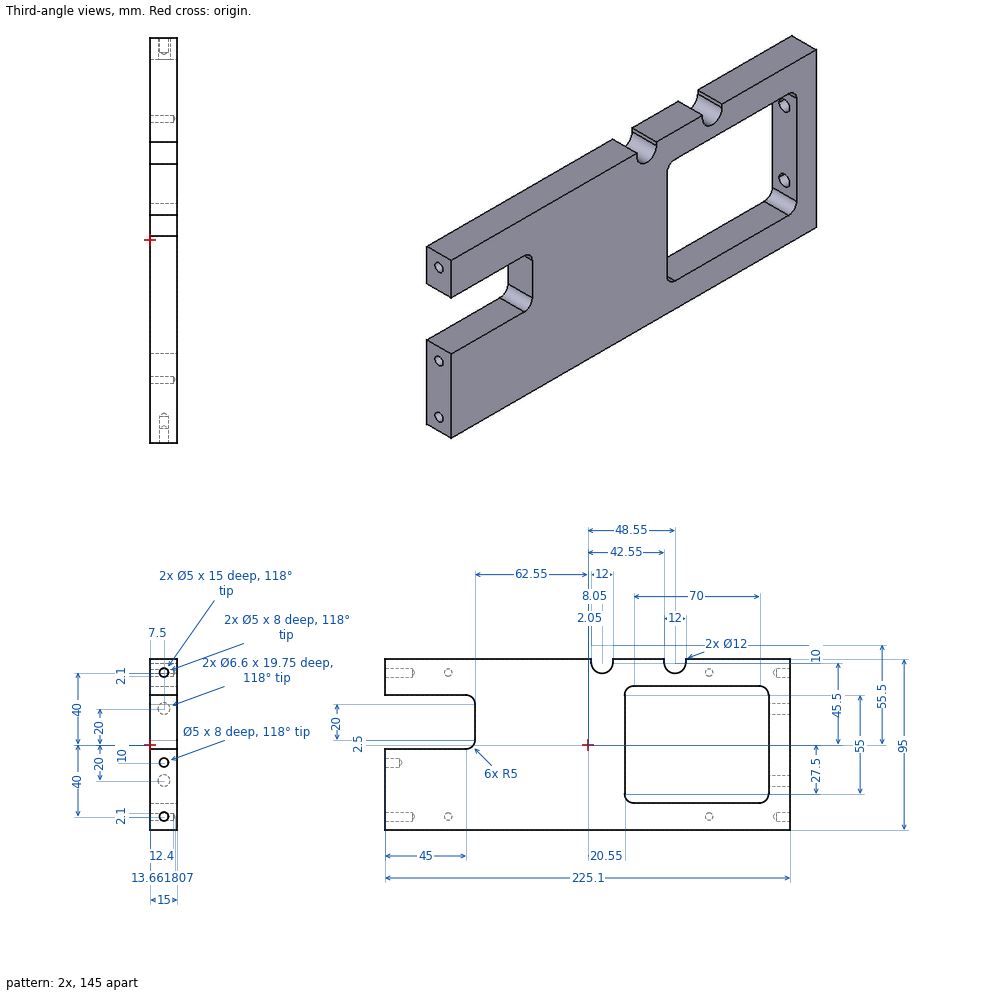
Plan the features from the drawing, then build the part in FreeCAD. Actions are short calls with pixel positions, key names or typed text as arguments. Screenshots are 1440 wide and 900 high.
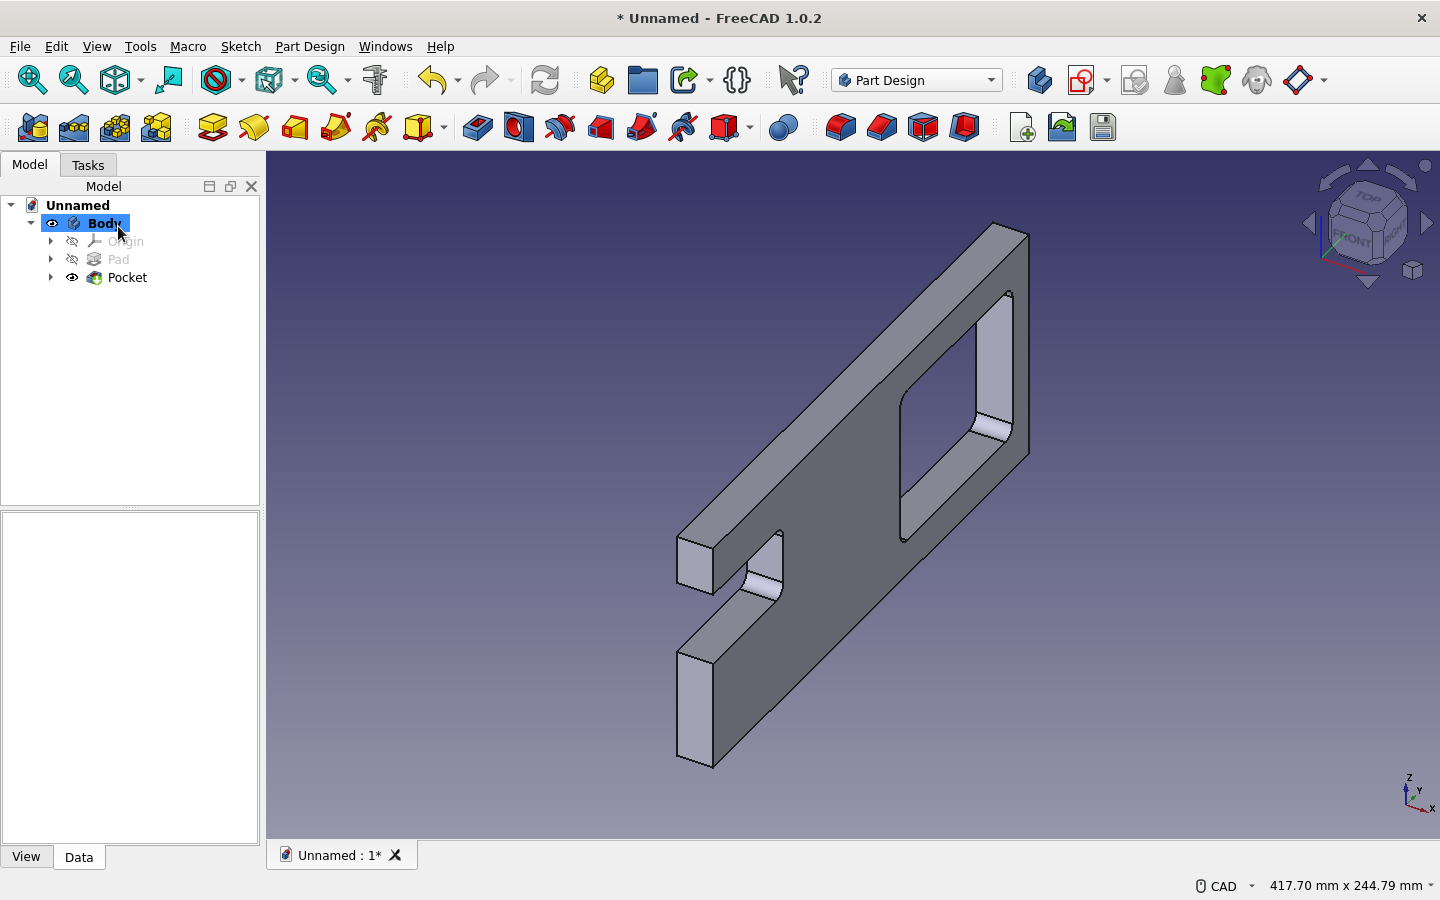
key(4)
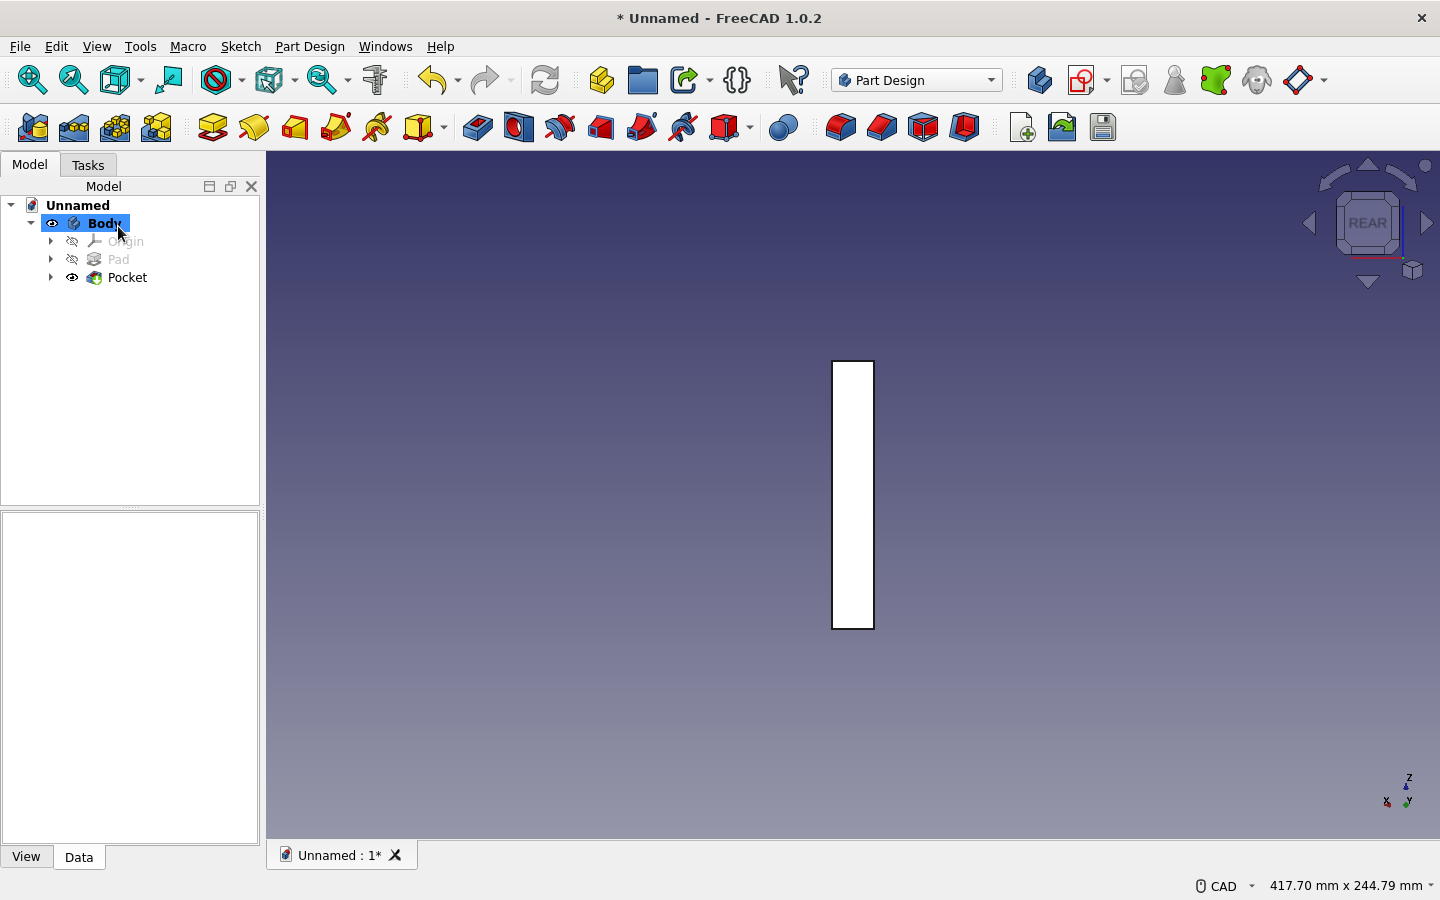
click(33, 80)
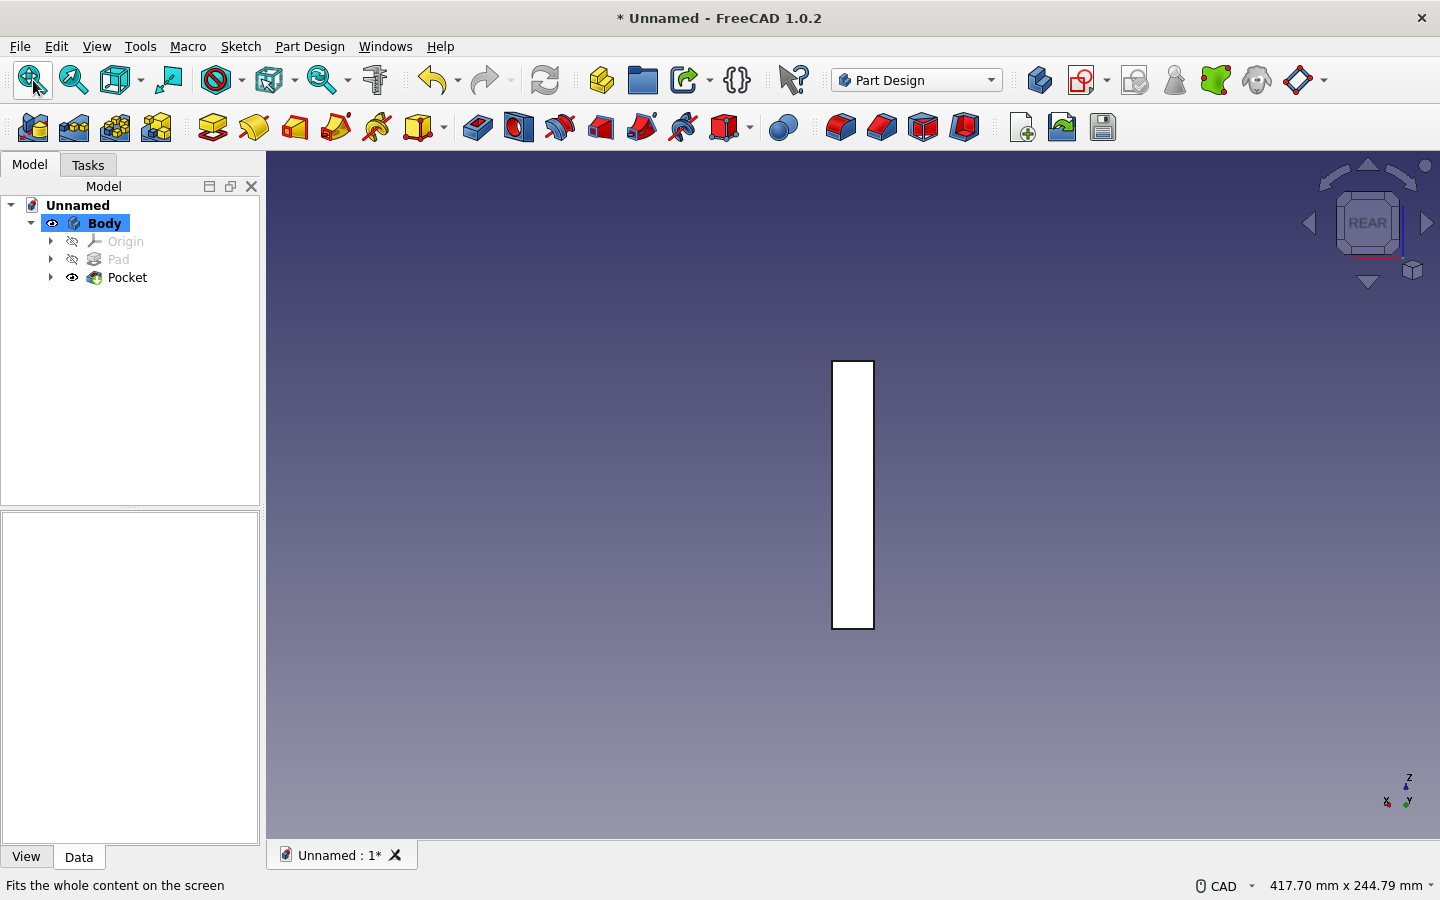
click(853, 494)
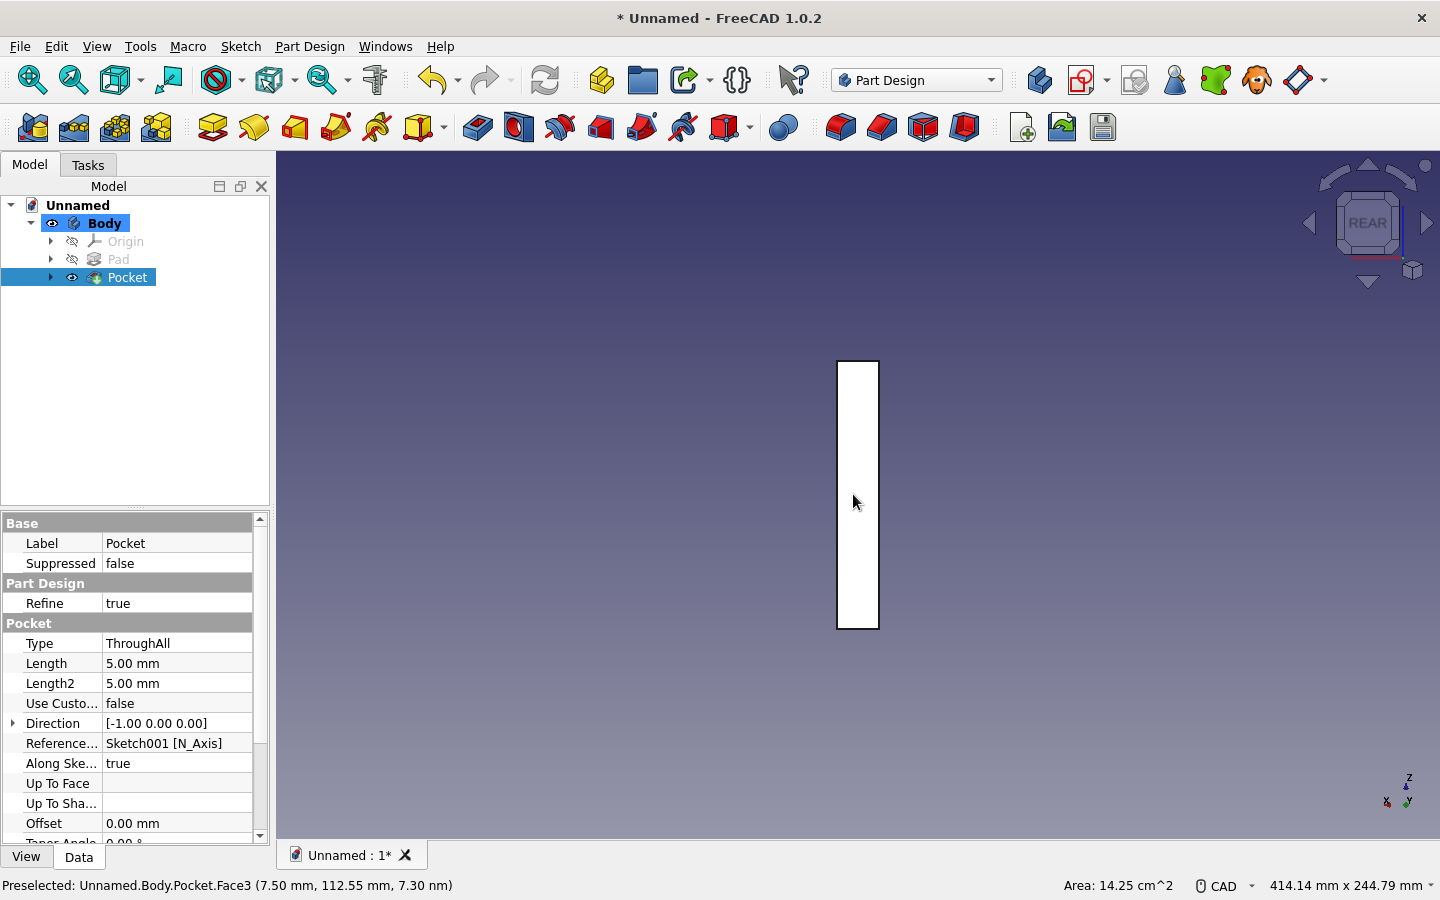
click(1080, 80)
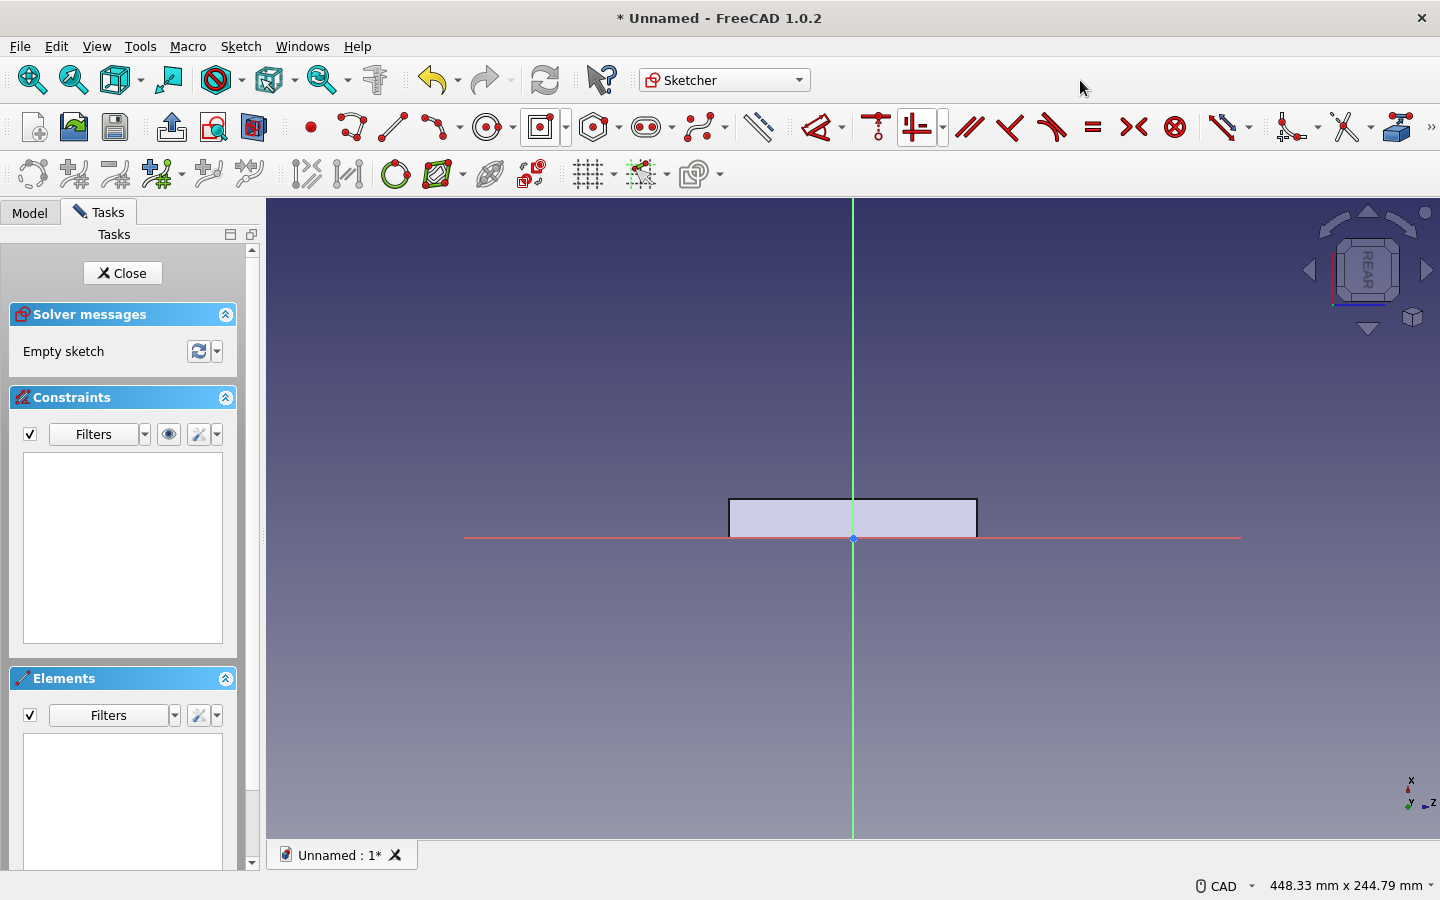
scroll(867, 525, up, 9)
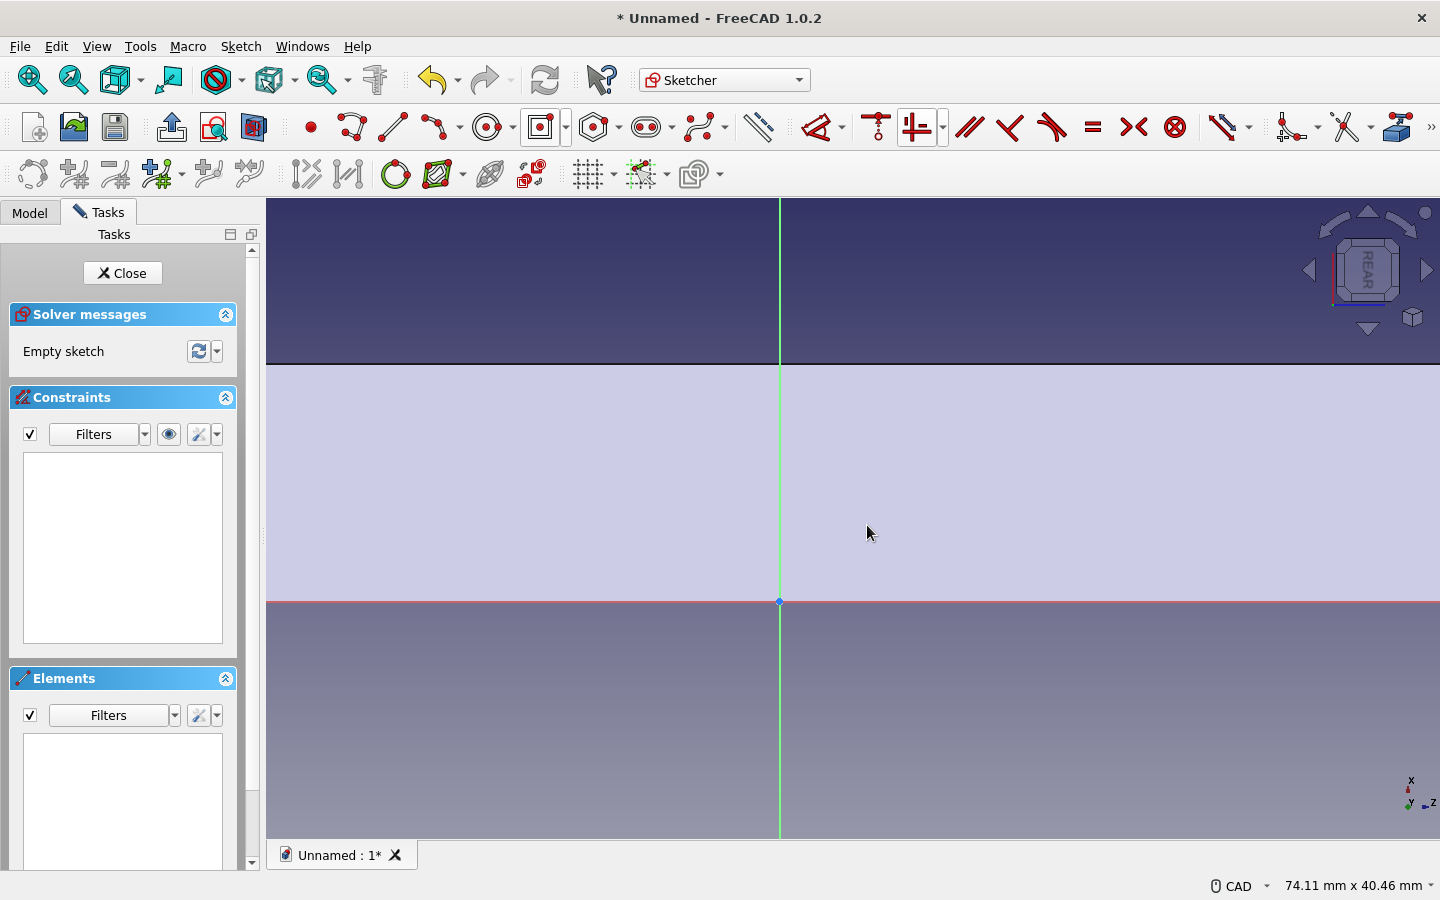
click(486, 128)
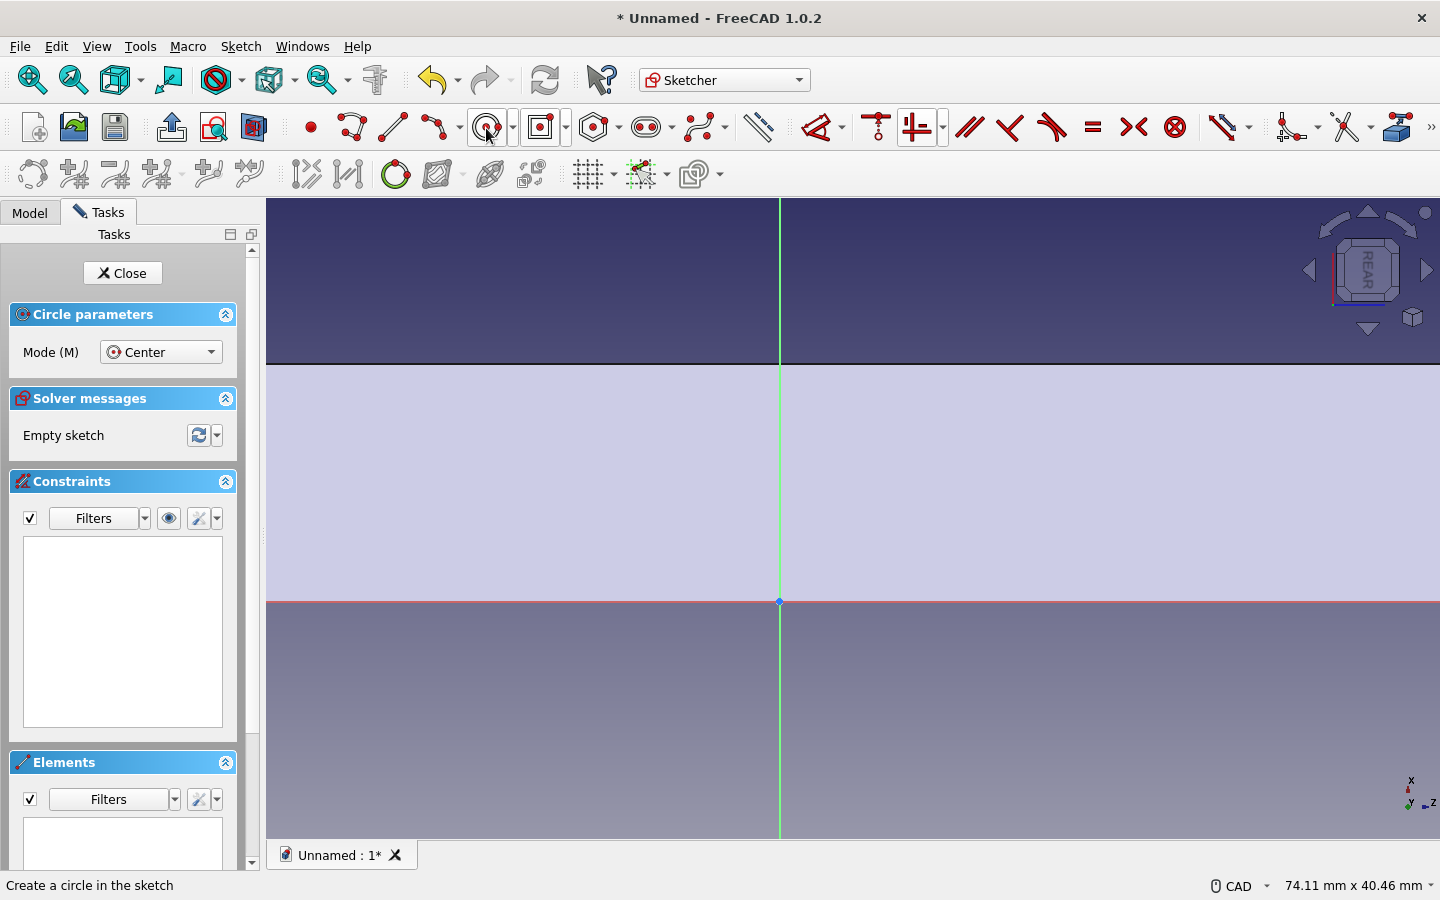
click(1097, 483)
move(1134, 446)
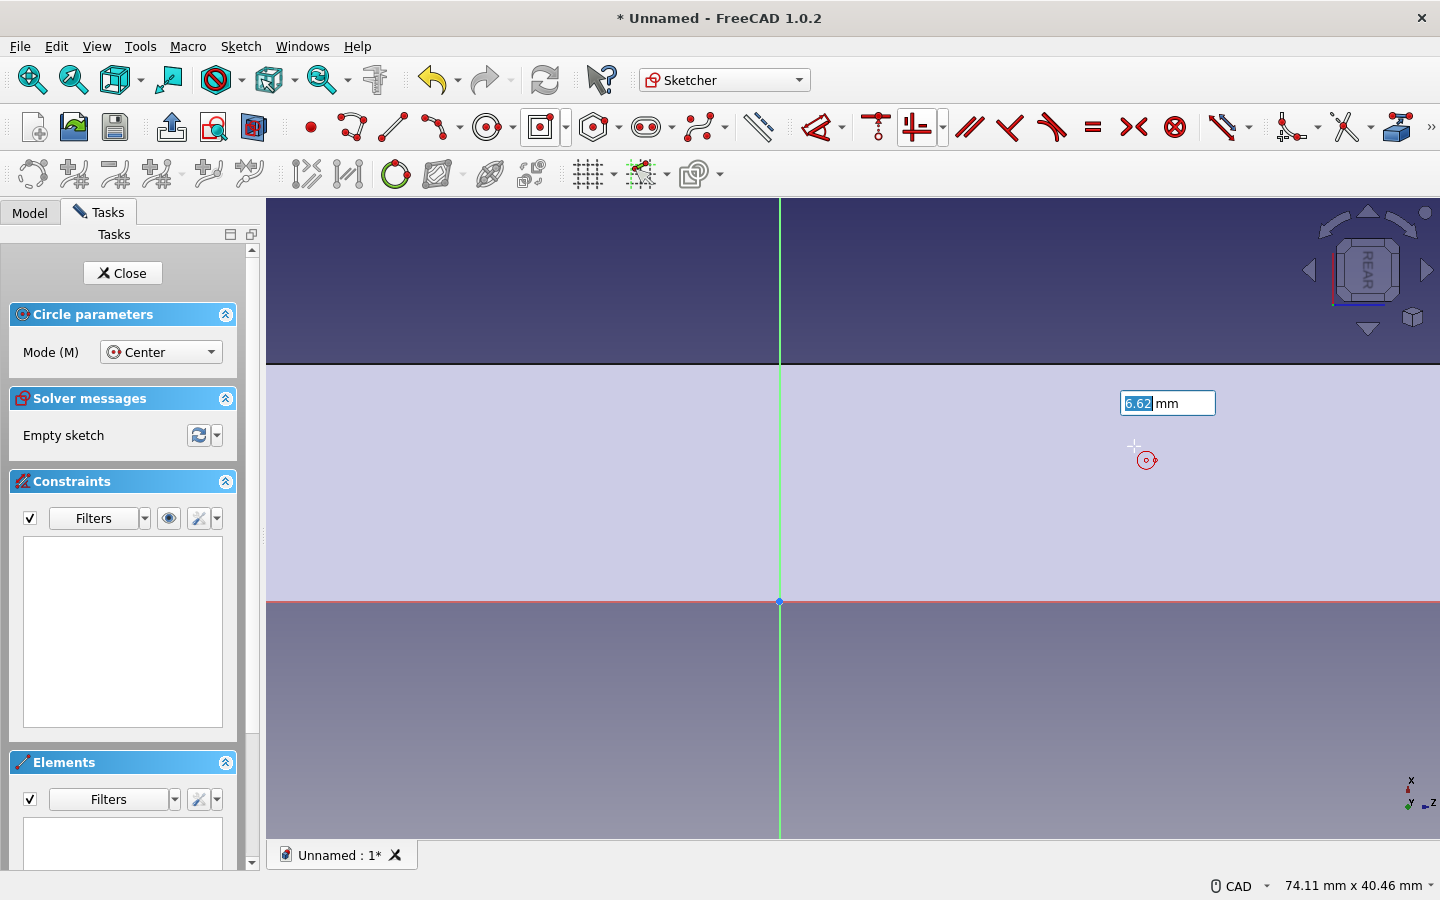
text(6.6)
key(Return)